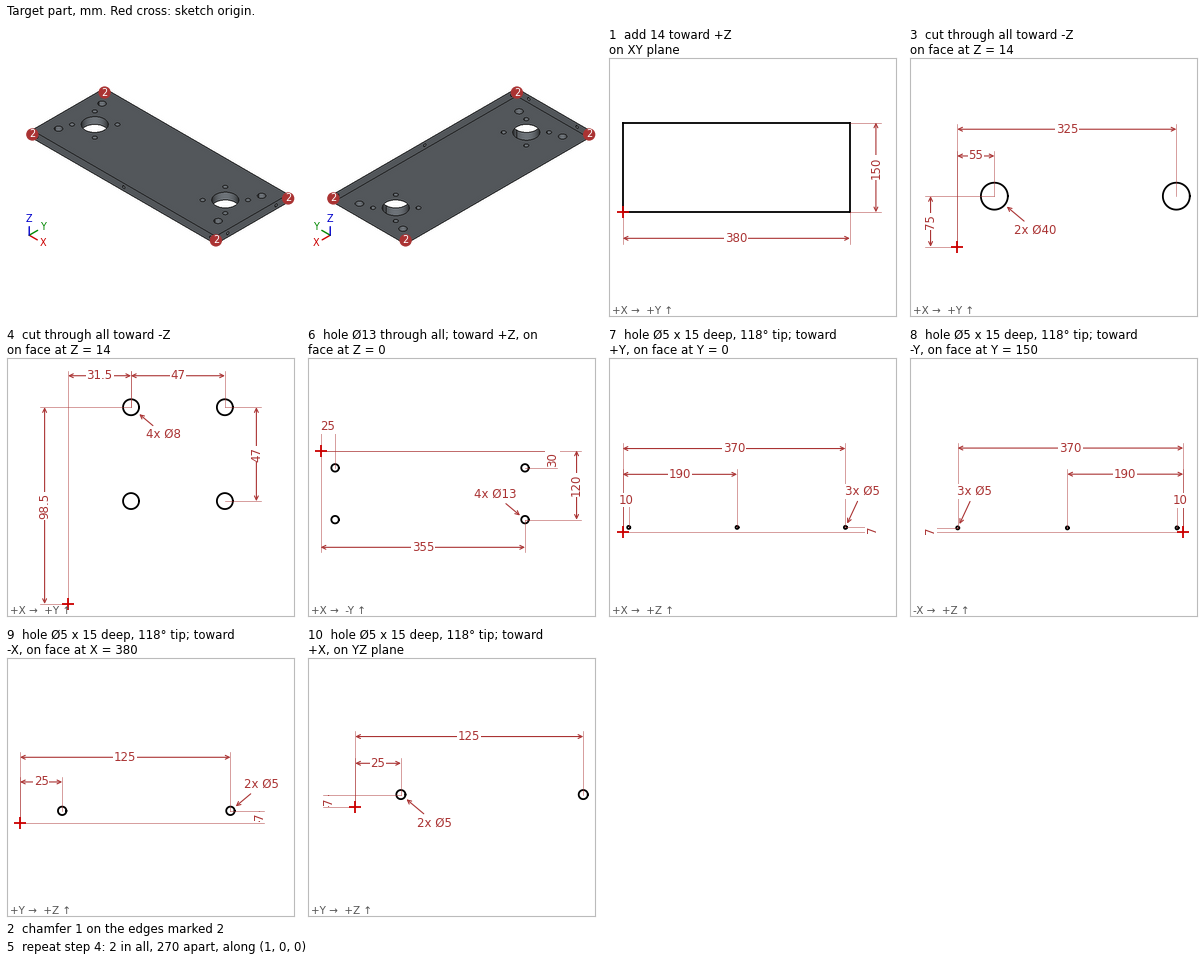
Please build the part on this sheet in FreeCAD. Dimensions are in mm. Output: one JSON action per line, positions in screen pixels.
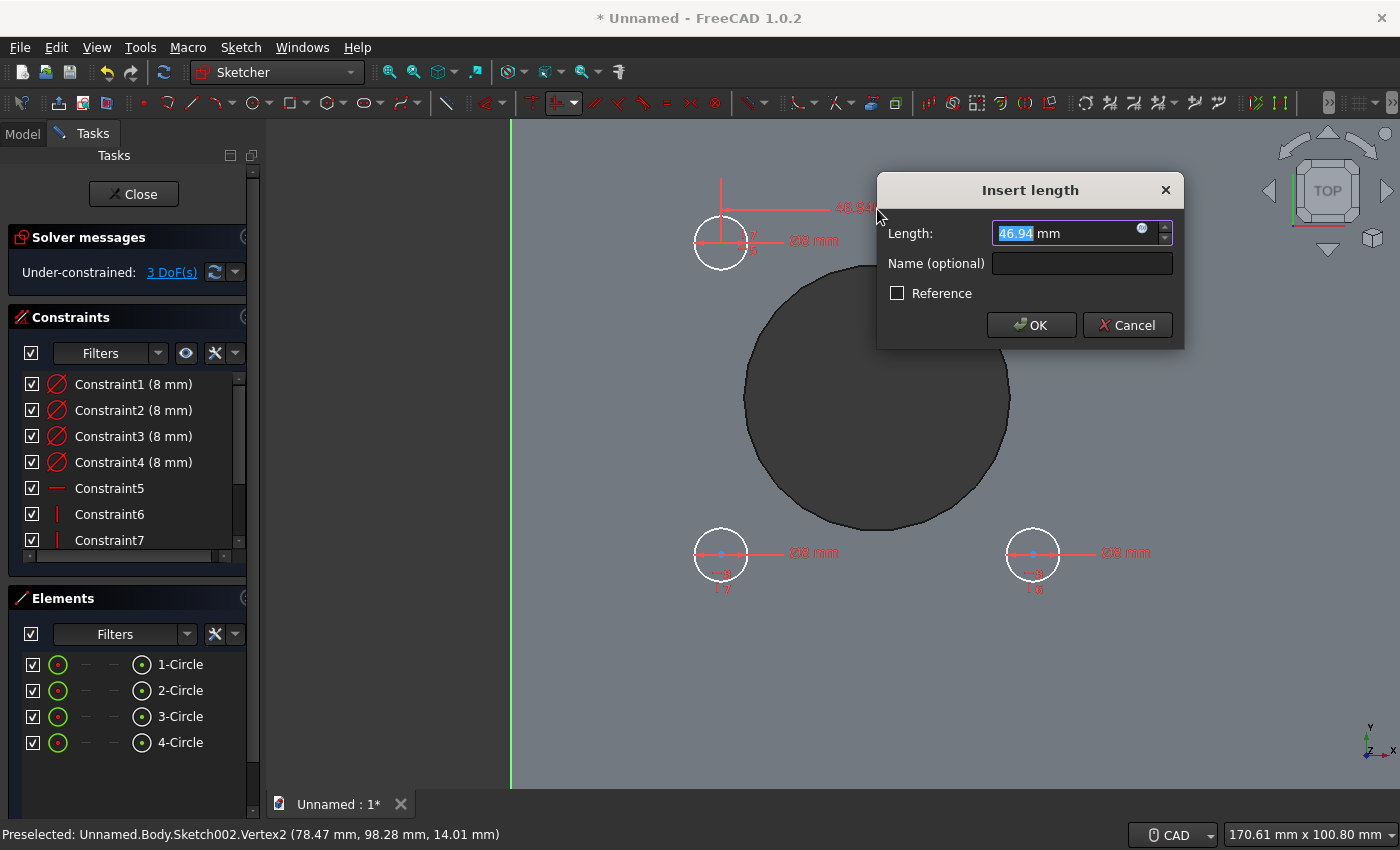
{"action": "type", "text": "47"}
{"action": "key", "text": "Return"}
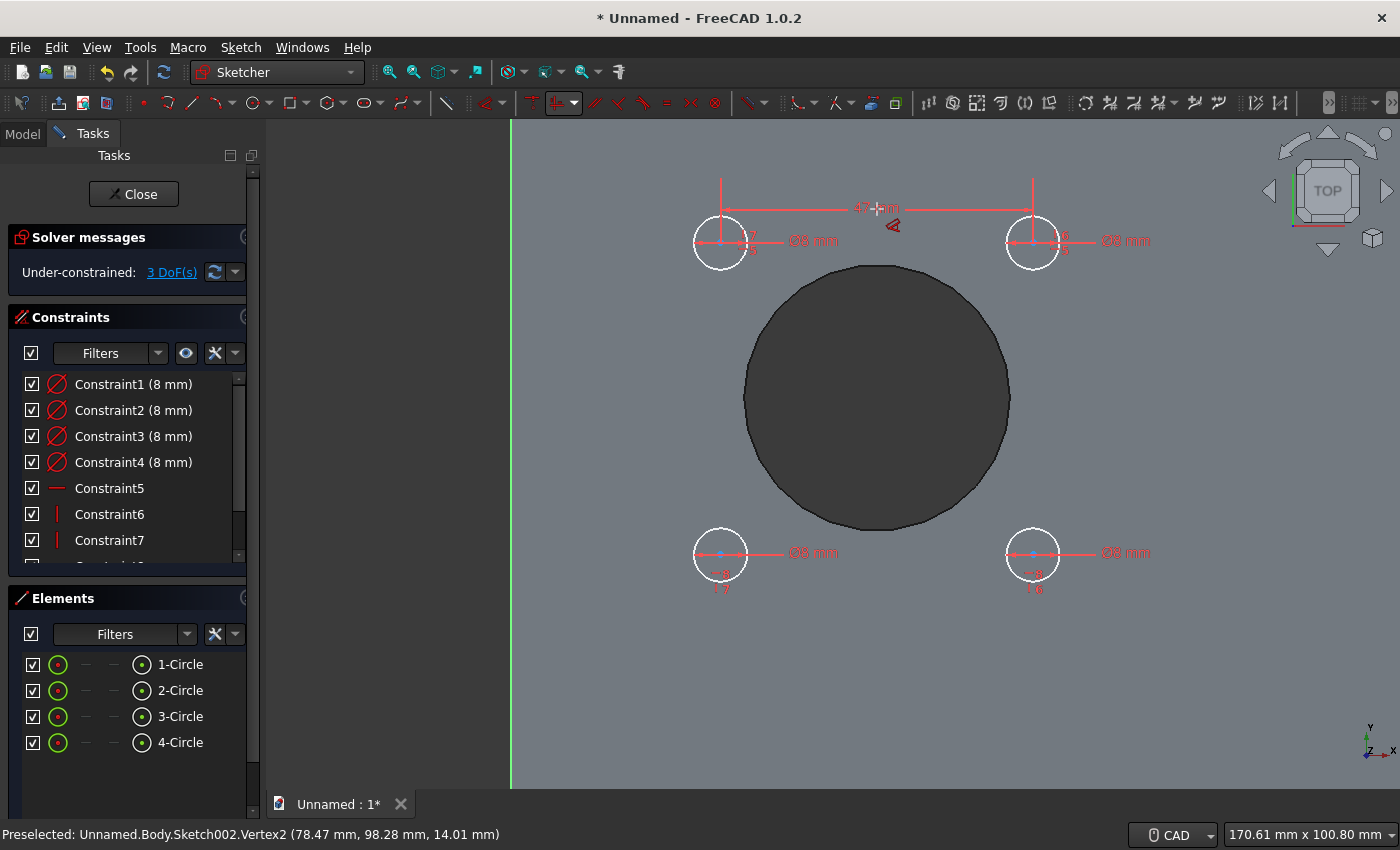
{"action": "left_click", "coordinate": [1033, 243]}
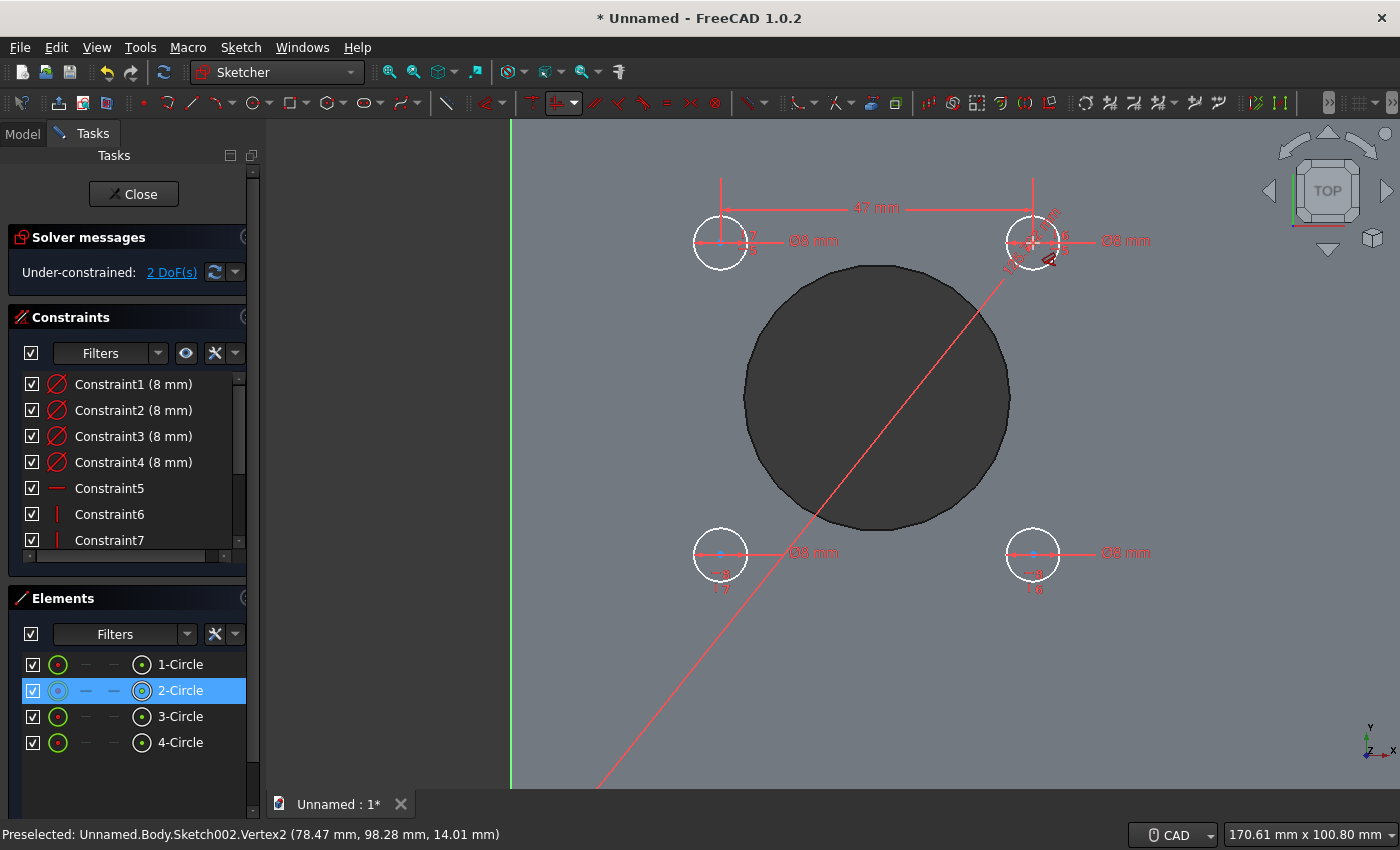
{"action": "left_click", "coordinate": [1033, 555]}
{"action": "left_click", "coordinate": [1067, 399]}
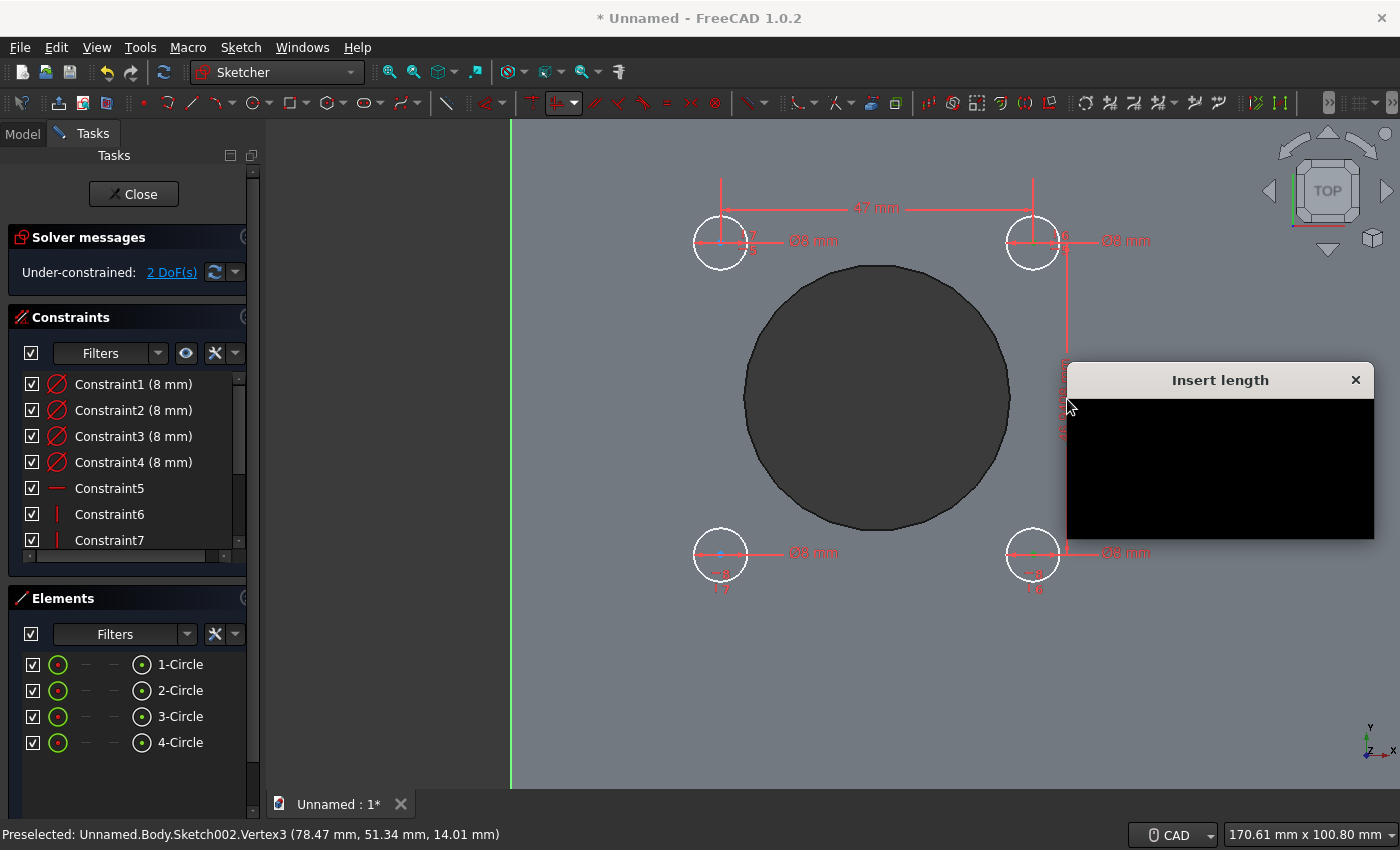
{"action": "type", "text": "47"}
{"action": "key", "text": "Return"}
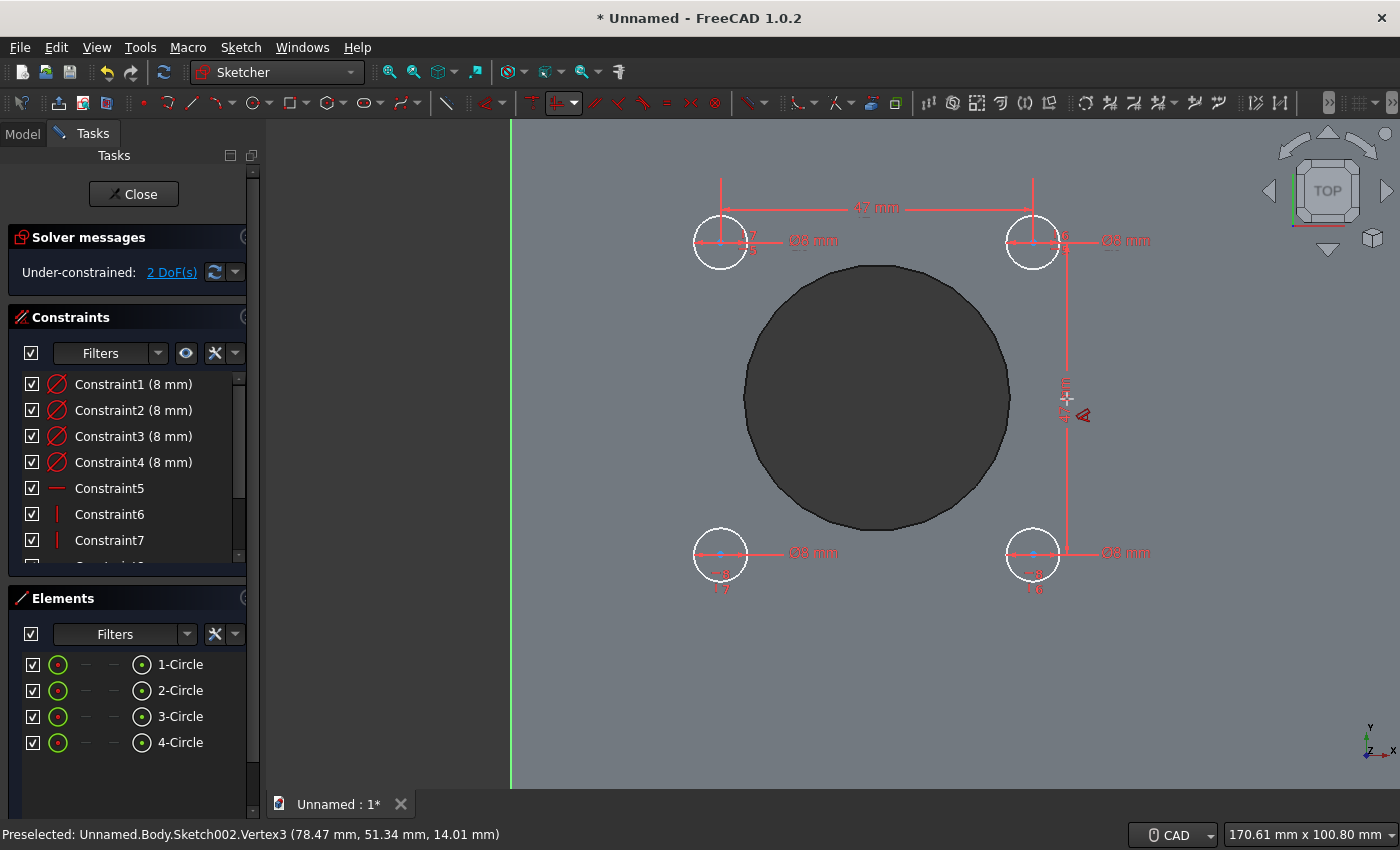
{"action": "left_click", "coordinate": [721, 243]}
{"action": "left_click", "coordinate": [616, 209]}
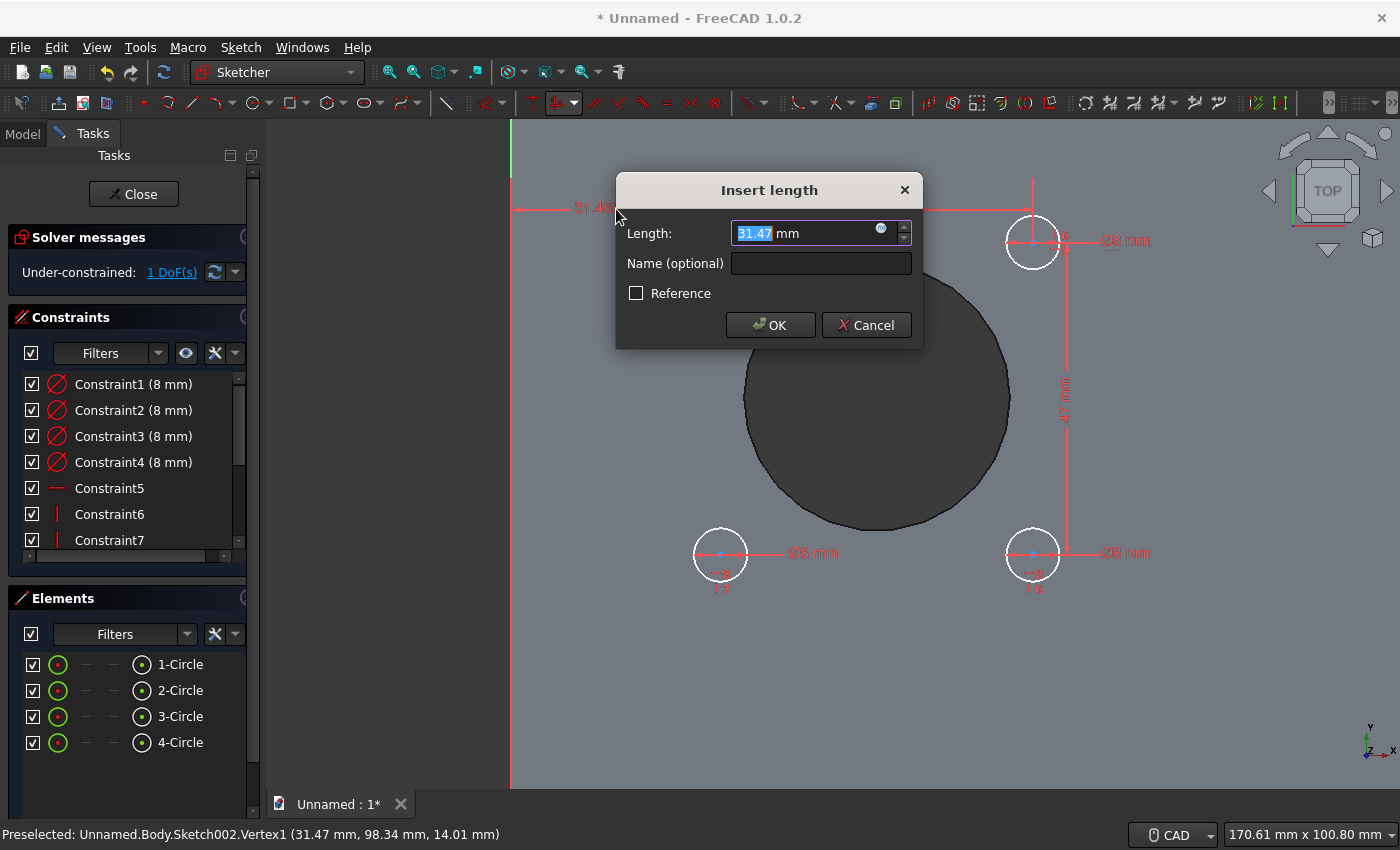
{"action": "type", "text": "31.5"}
{"action": "key", "text": "Return"}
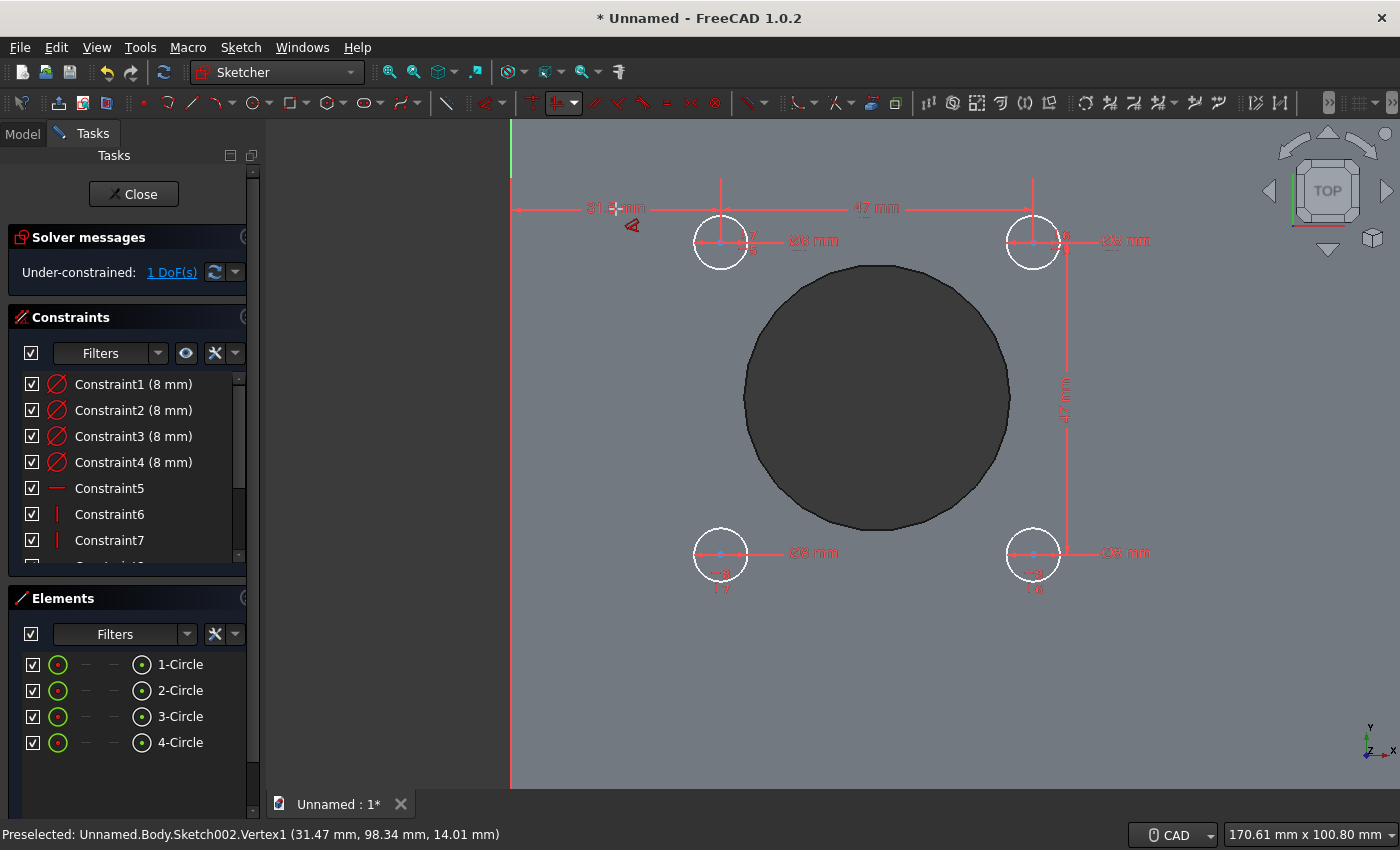
{"action": "left_click", "coordinate": [721, 243]}
{"action": "left_click", "coordinate": [477, 502]}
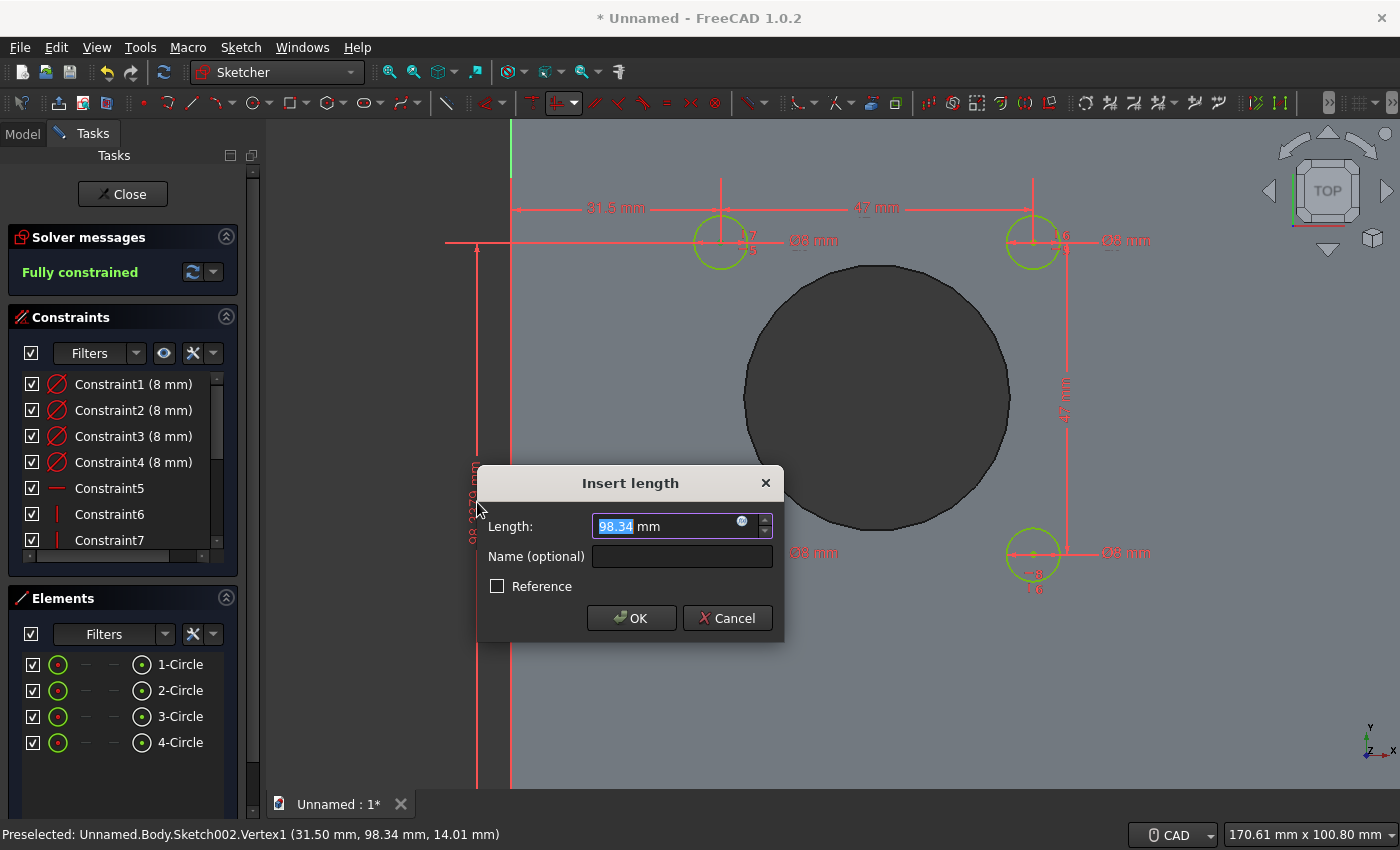
{"action": "type", "text": "98.5"}
{"action": "key", "text": "Return"}
{"action": "key", "text": "Escape"}